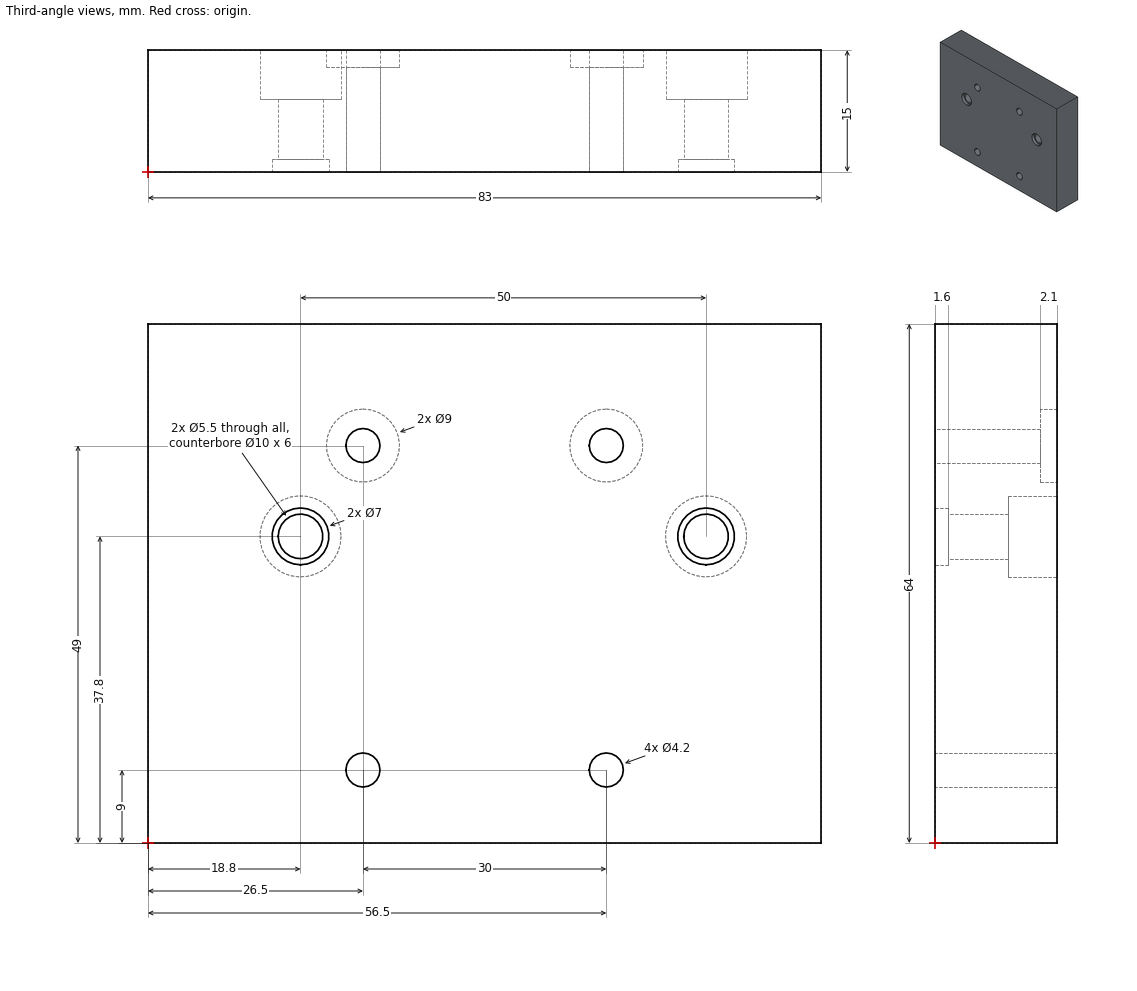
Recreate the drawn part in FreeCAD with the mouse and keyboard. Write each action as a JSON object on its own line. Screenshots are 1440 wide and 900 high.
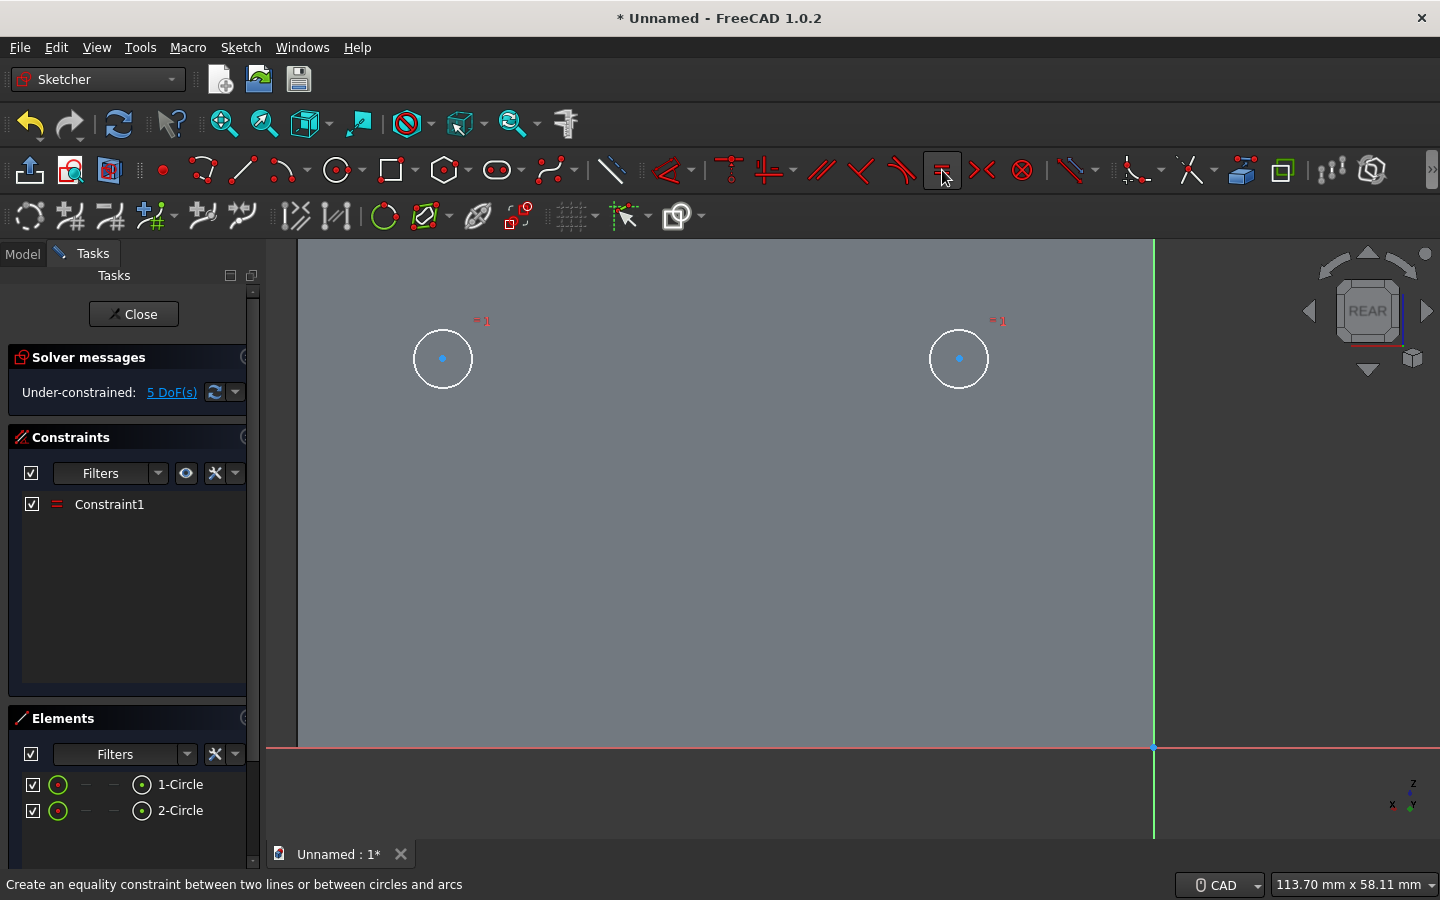
{"action": "left_click", "coordinate": [666, 170]}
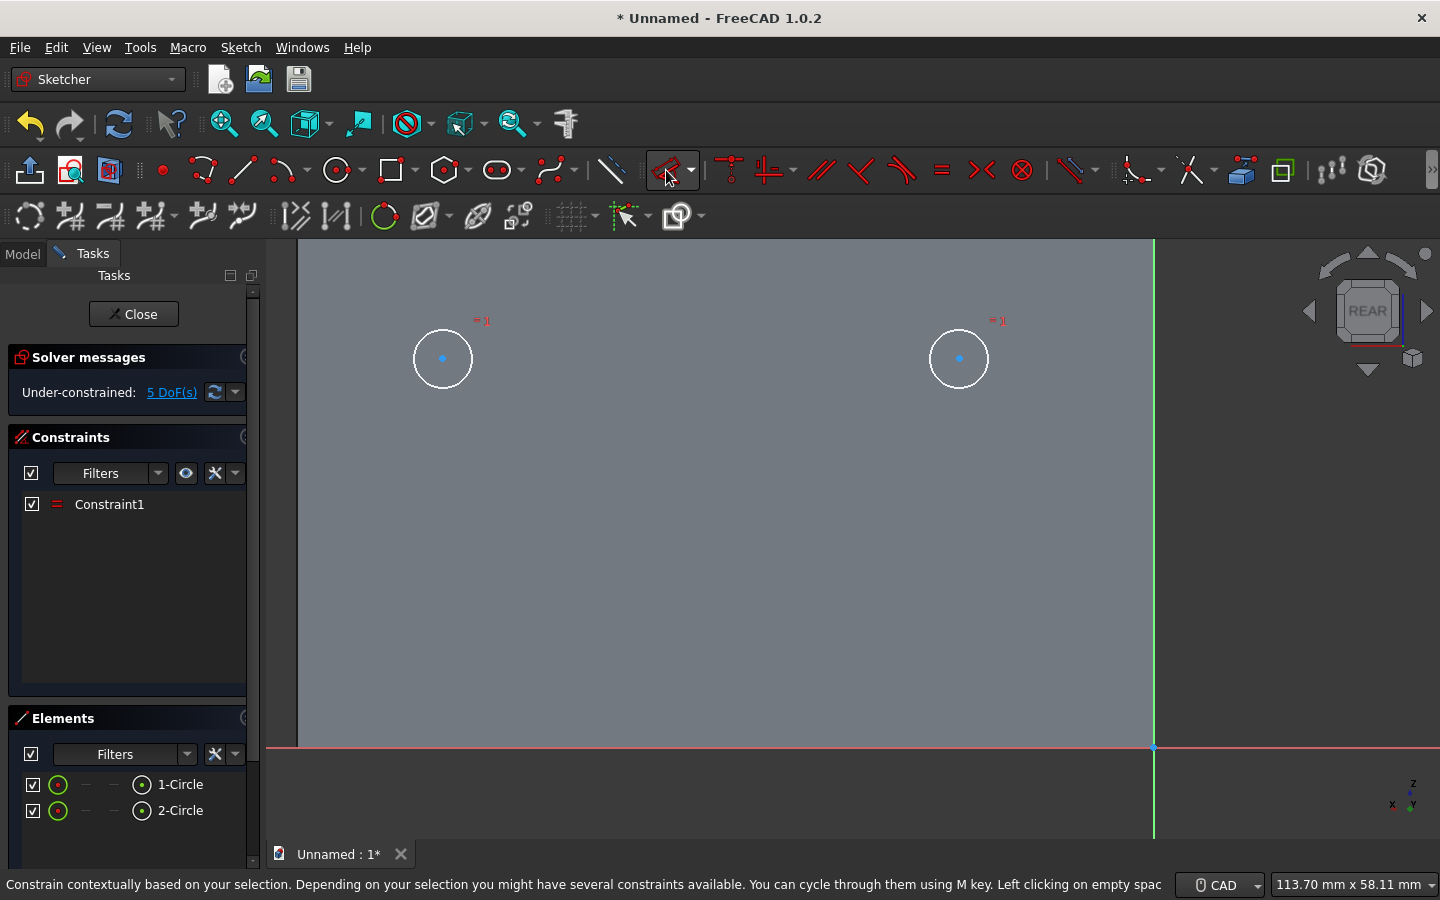
{"action": "left_click", "coordinate": [979, 338]}
{"action": "left_click", "coordinate": [1001, 315]}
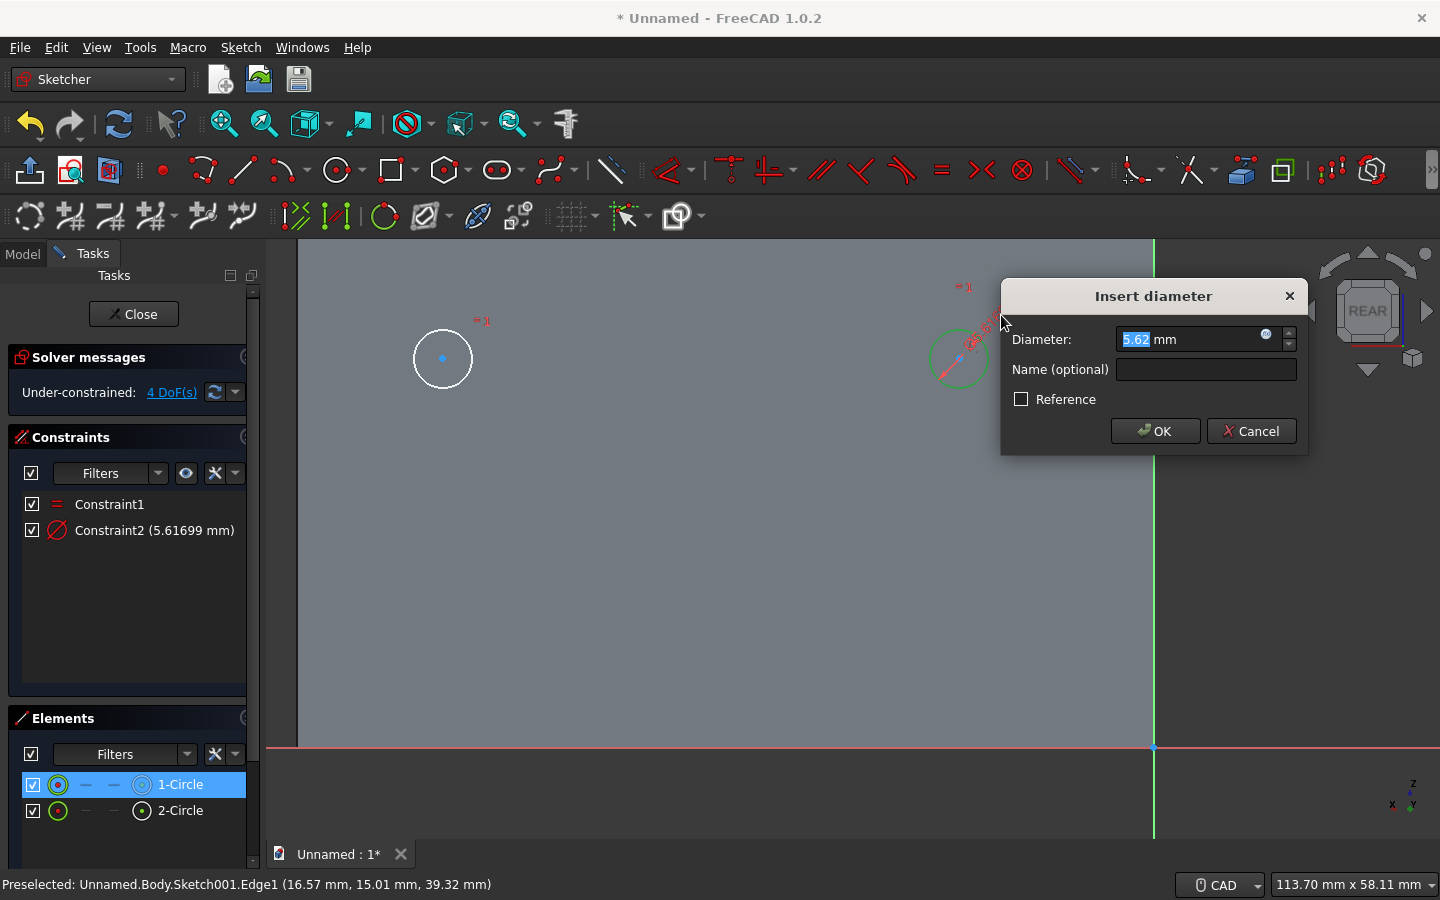
{"action": "type", "text": "5.5"}
{"action": "key", "text": "Return"}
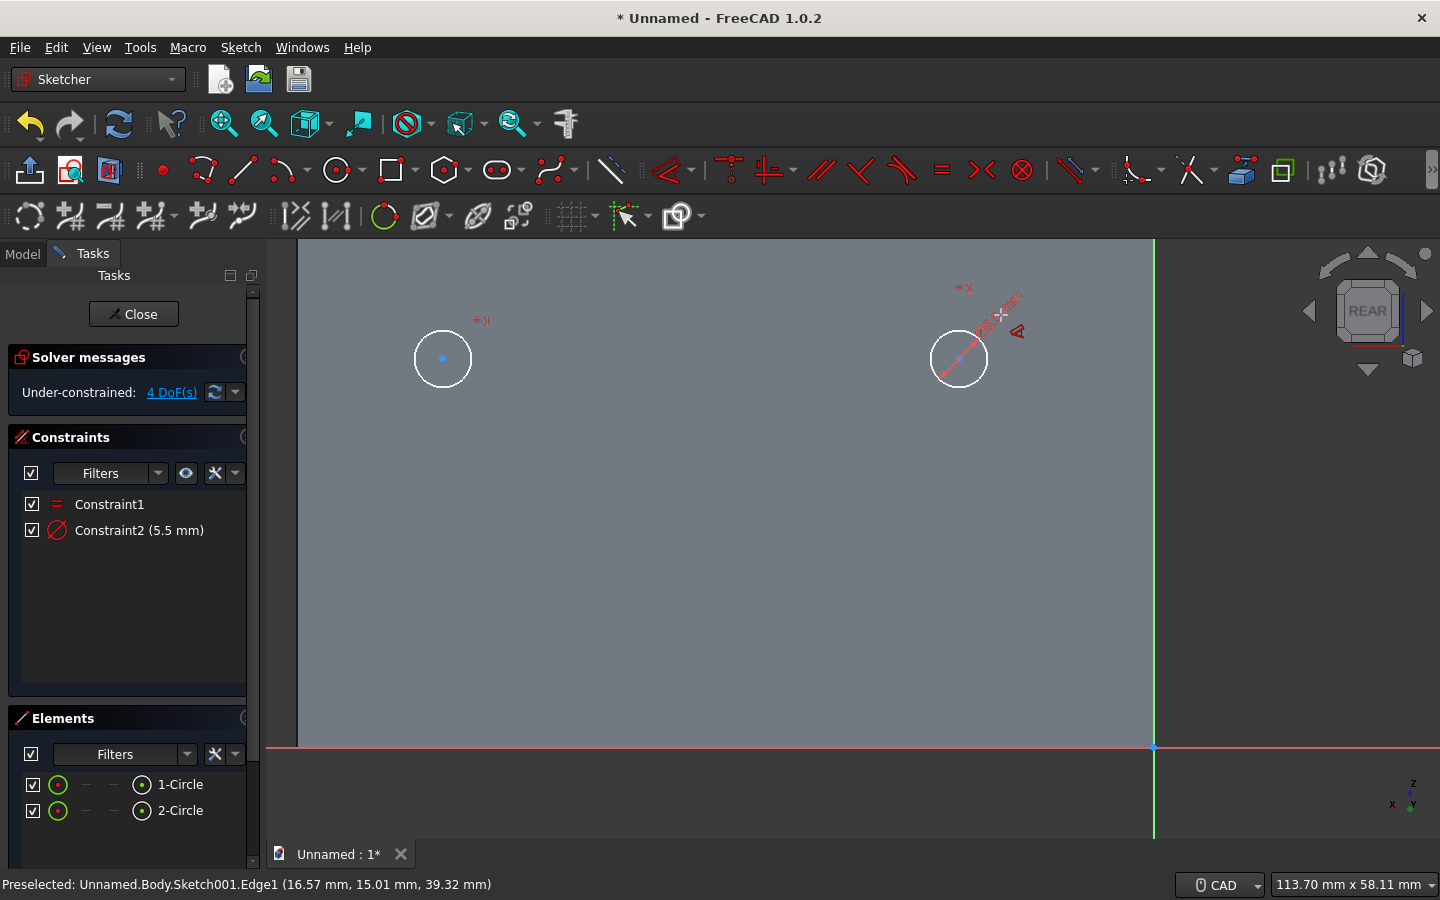
{"action": "left_click", "coordinate": [959, 359]}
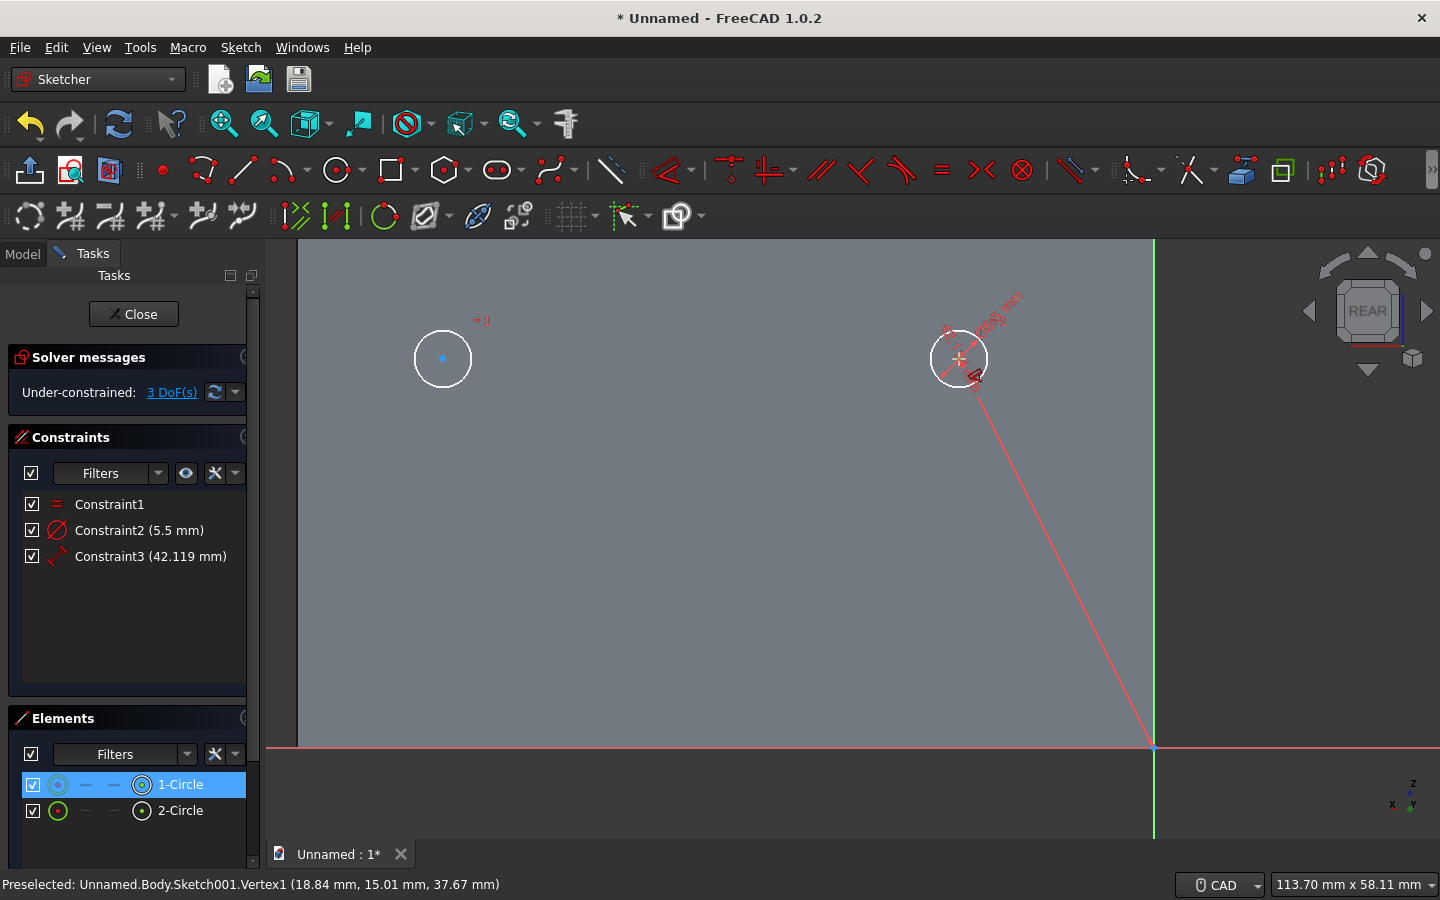
{"action": "left_click", "coordinate": [443, 359]}
{"action": "left_click", "coordinate": [701, 325]}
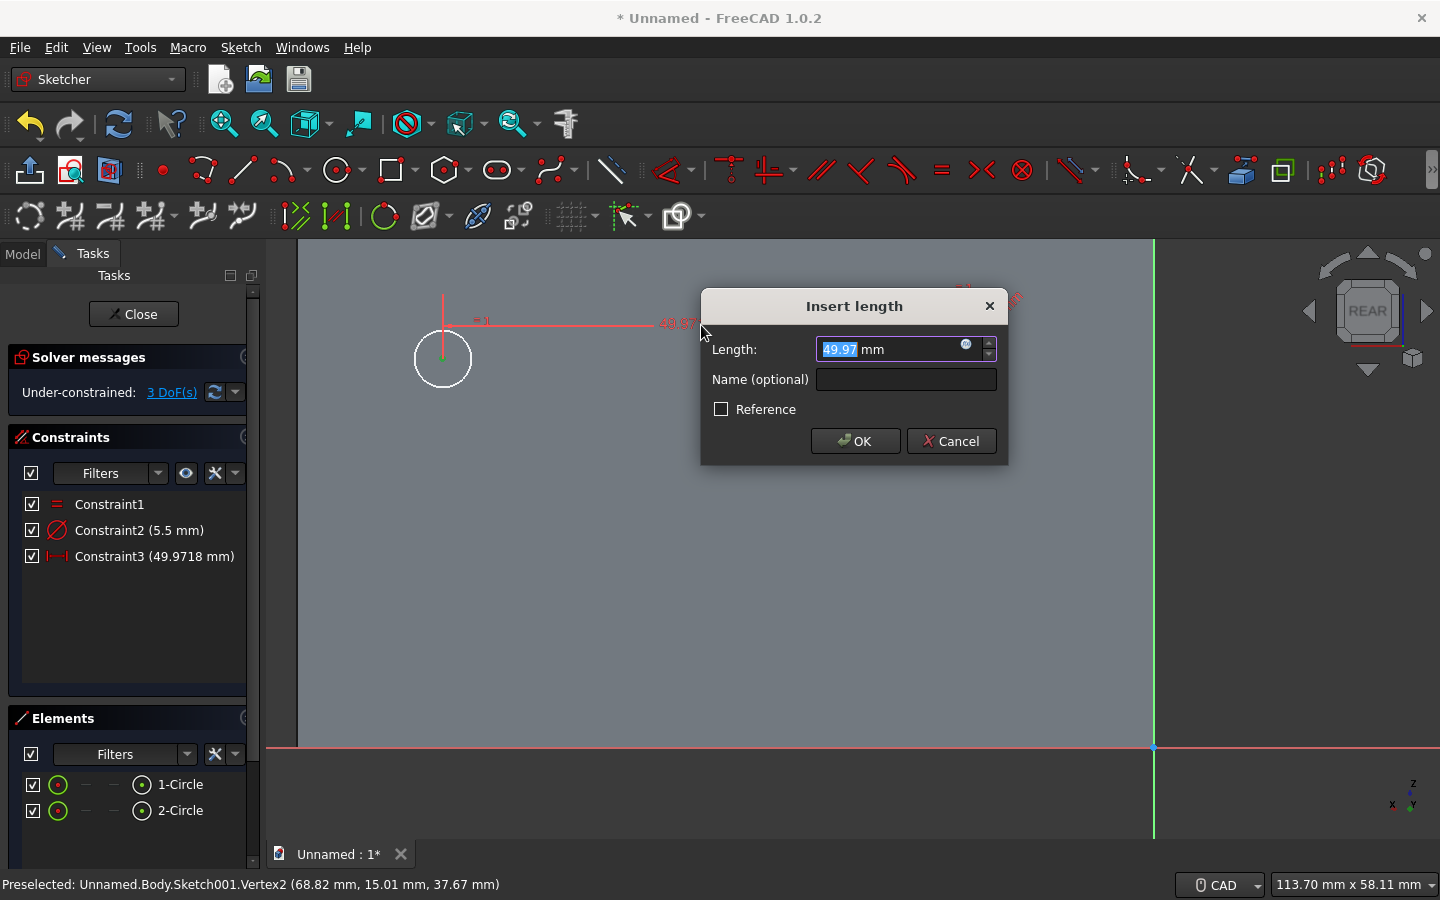
{"action": "type", "text": "50"}
{"action": "key", "text": "Return"}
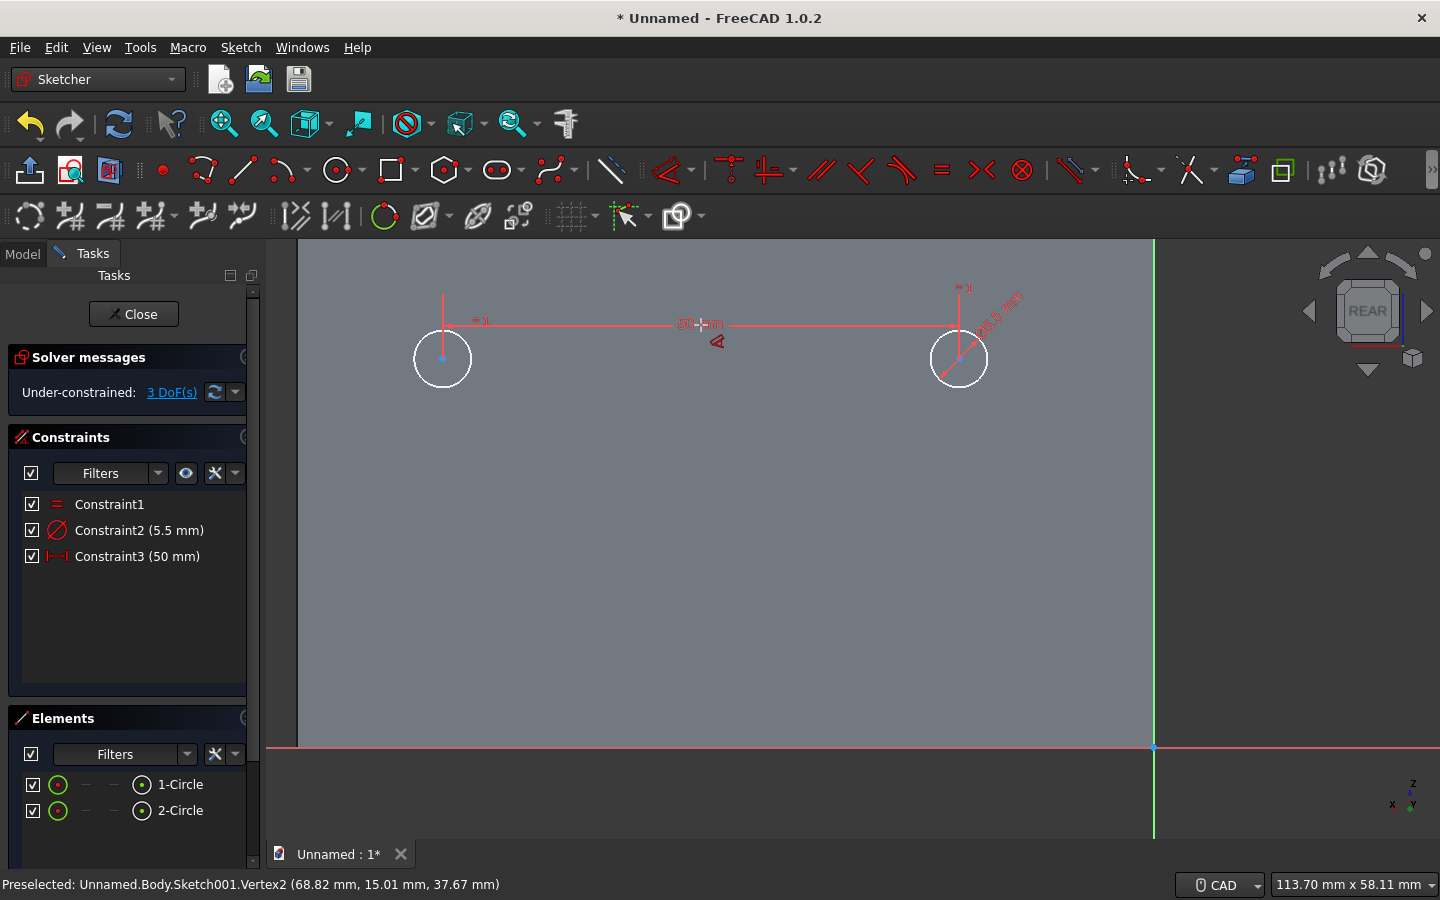
{"action": "left_click", "coordinate": [959, 359]}
{"action": "left_click", "coordinate": [1056, 782]}